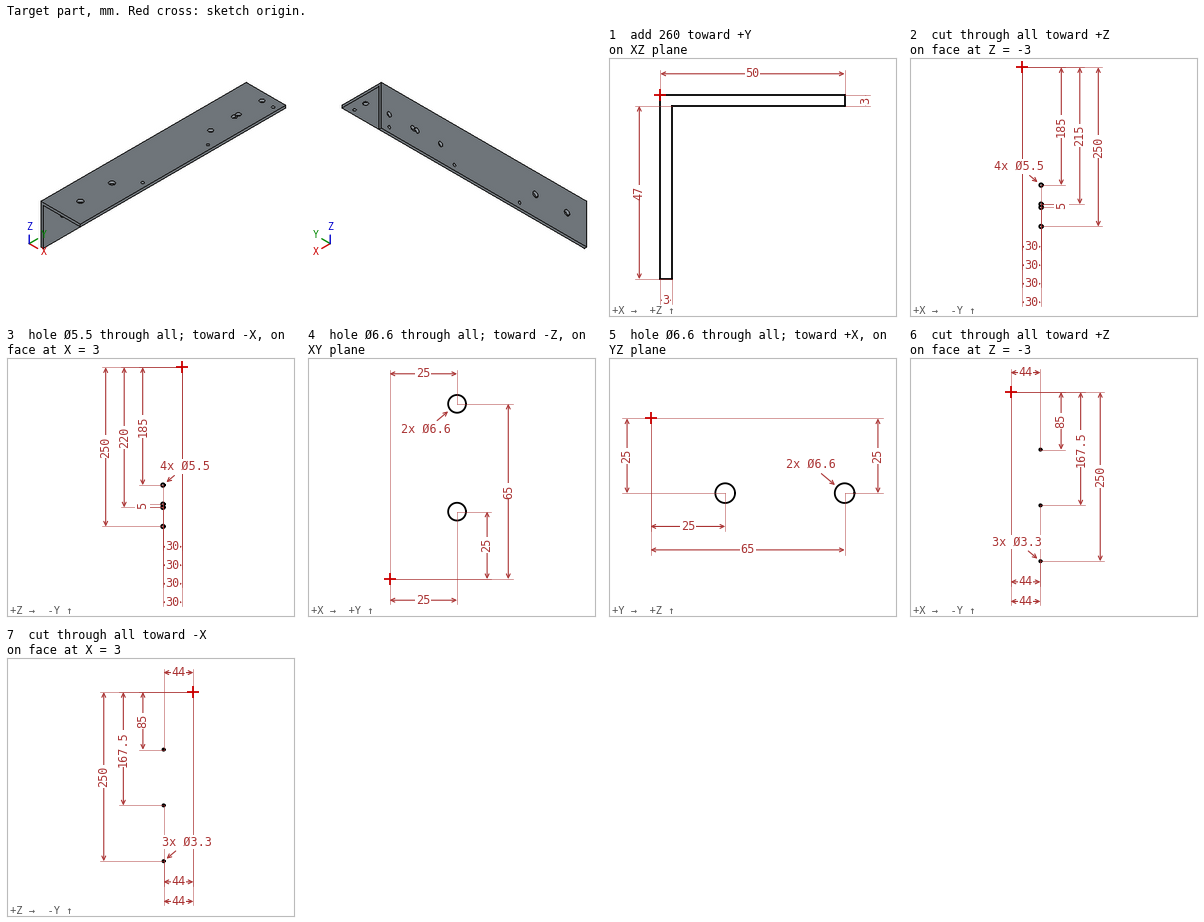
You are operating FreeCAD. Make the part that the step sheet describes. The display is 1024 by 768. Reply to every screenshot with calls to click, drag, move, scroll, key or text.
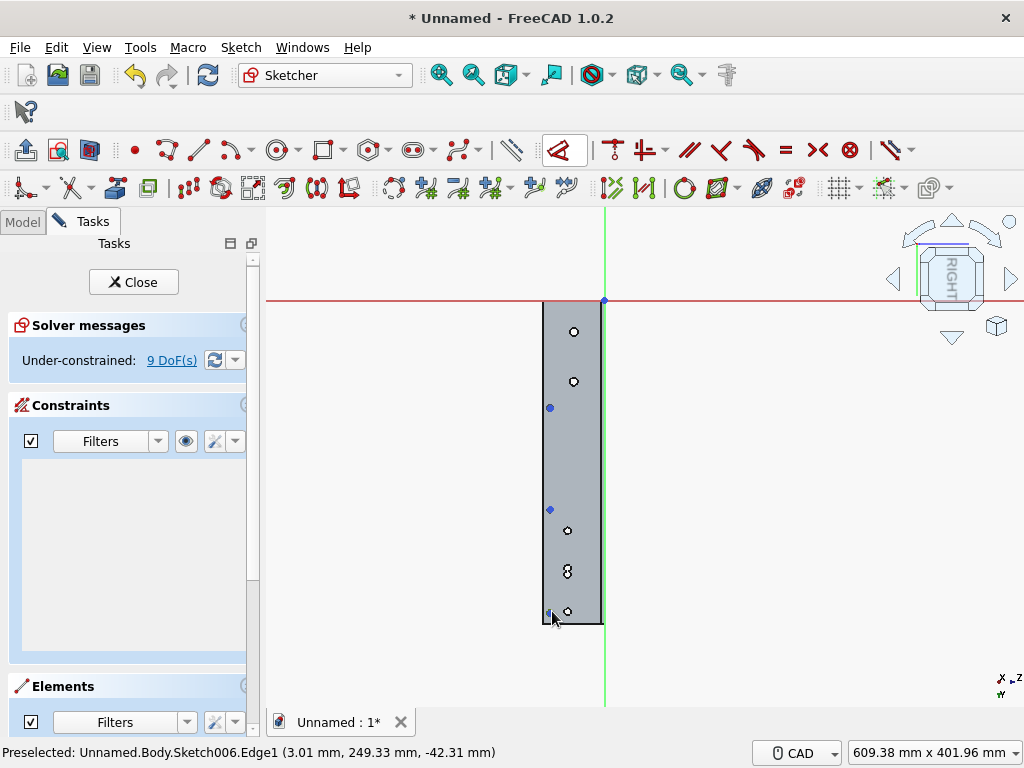
scroll(552, 508, up, 8)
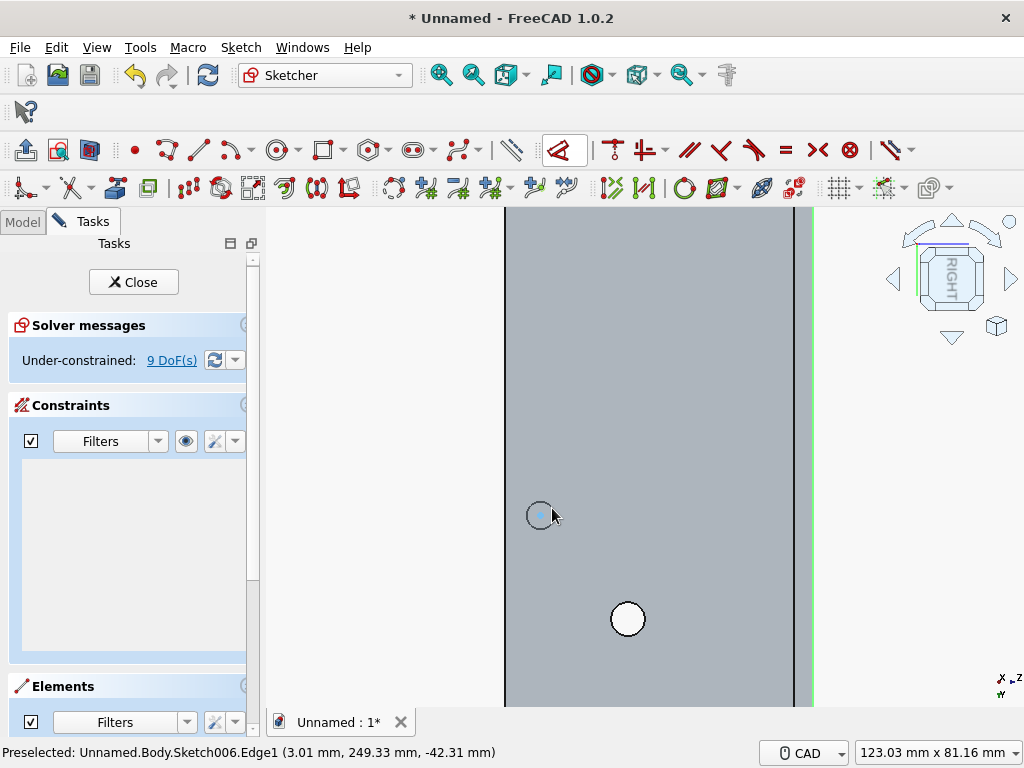
click(550, 506)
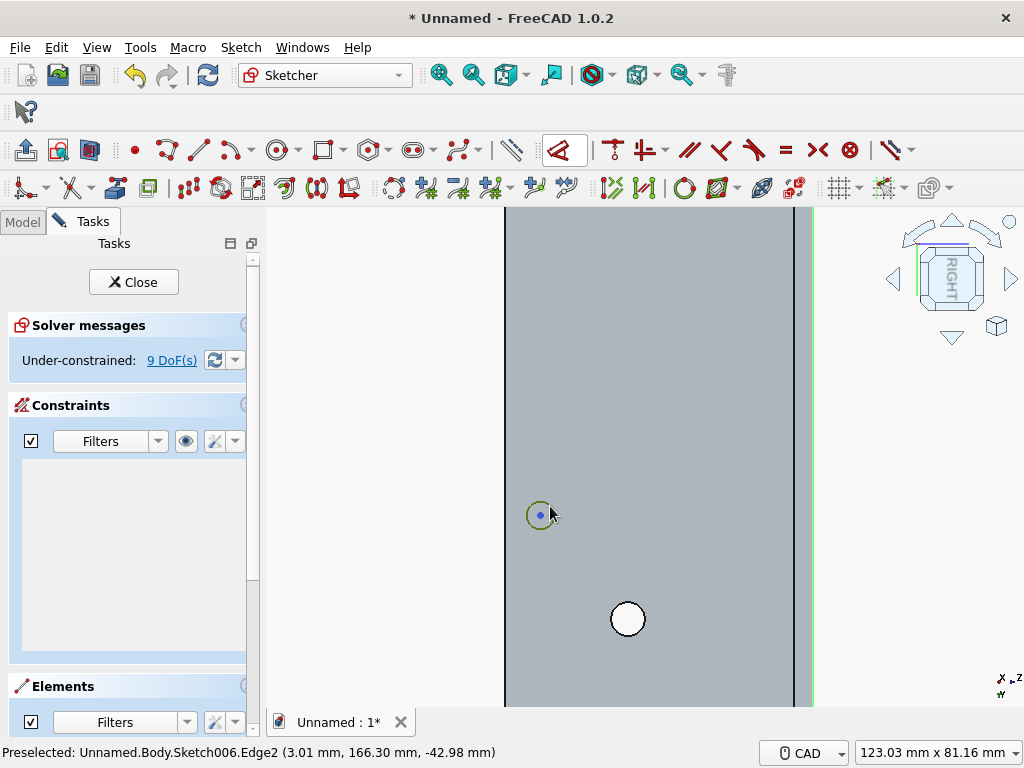
scroll(552, 508, down, 8)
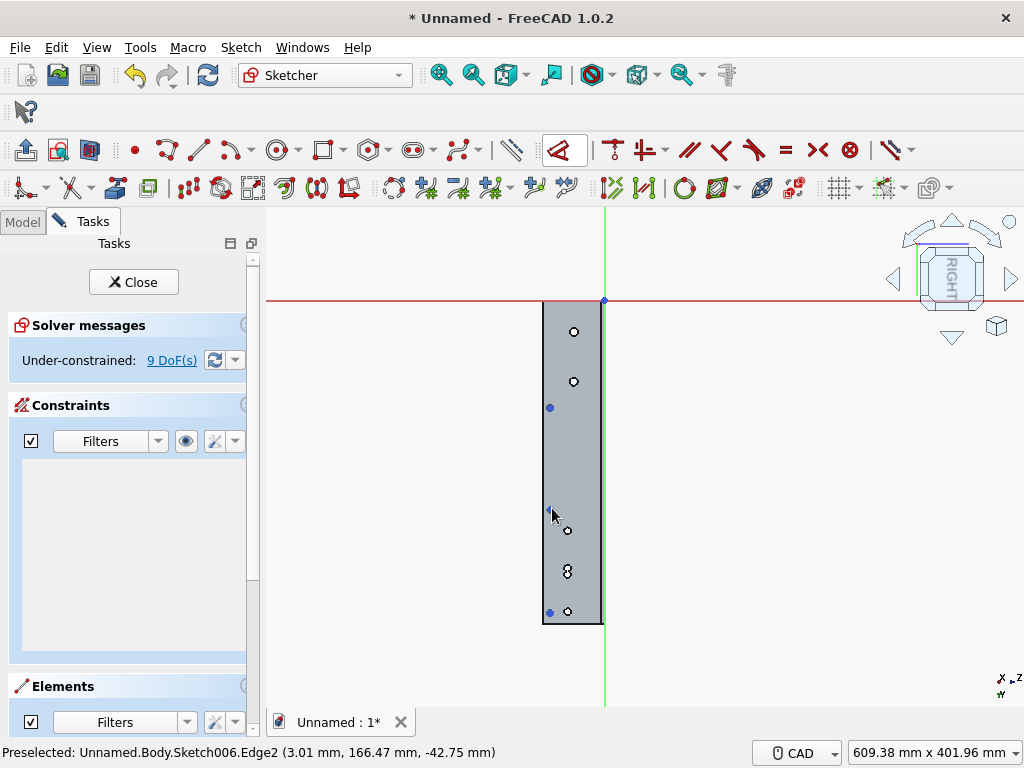
scroll(552, 406, up, 8)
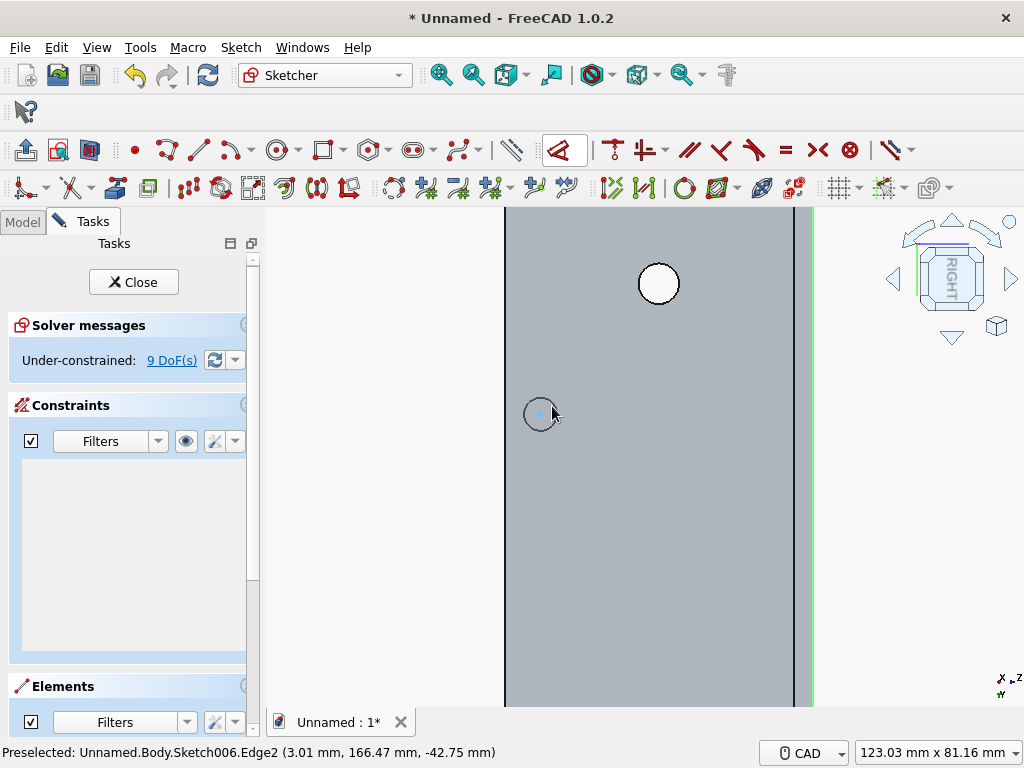
click(552, 403)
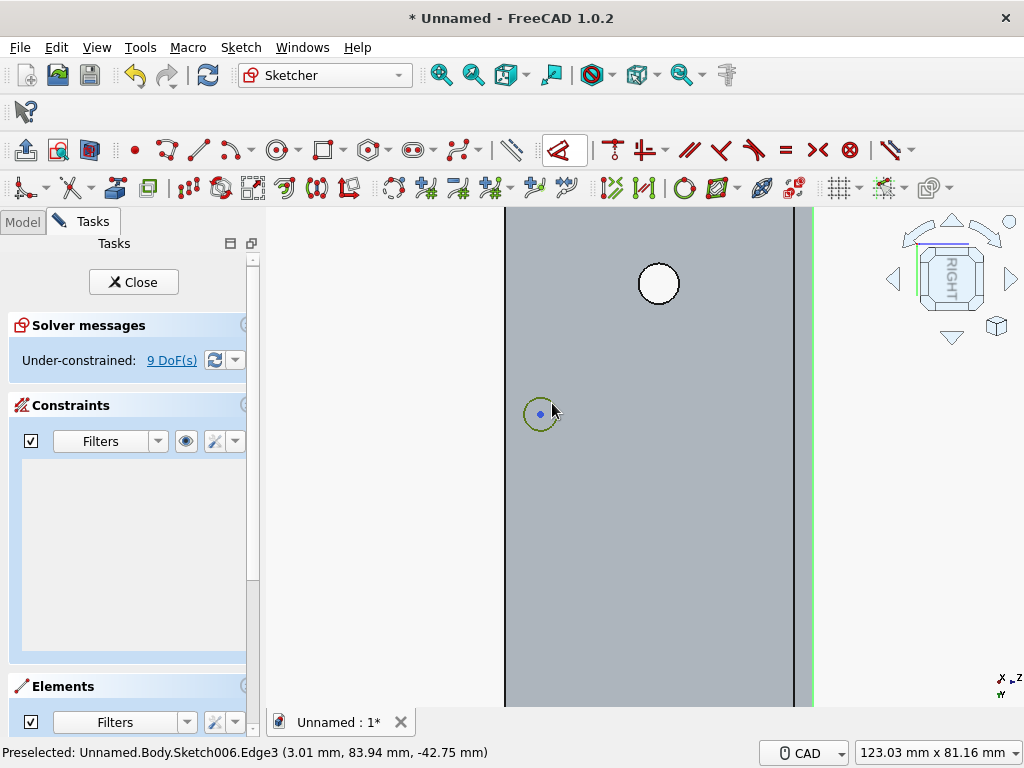
click(786, 150)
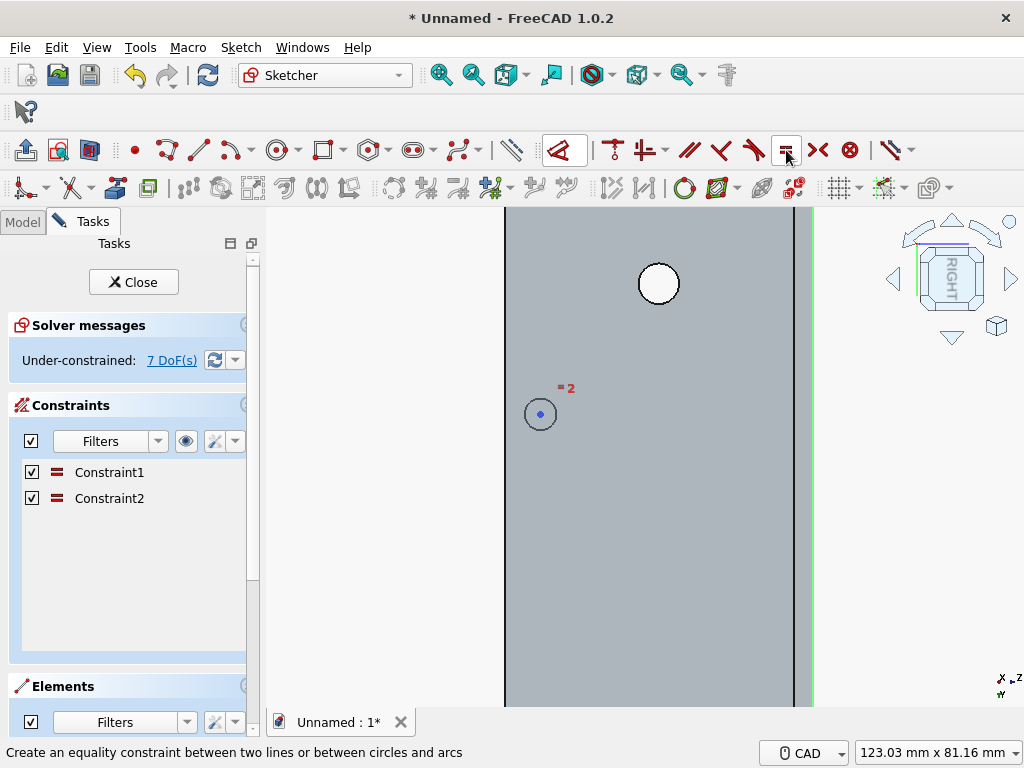
scroll(552, 406, down, 8)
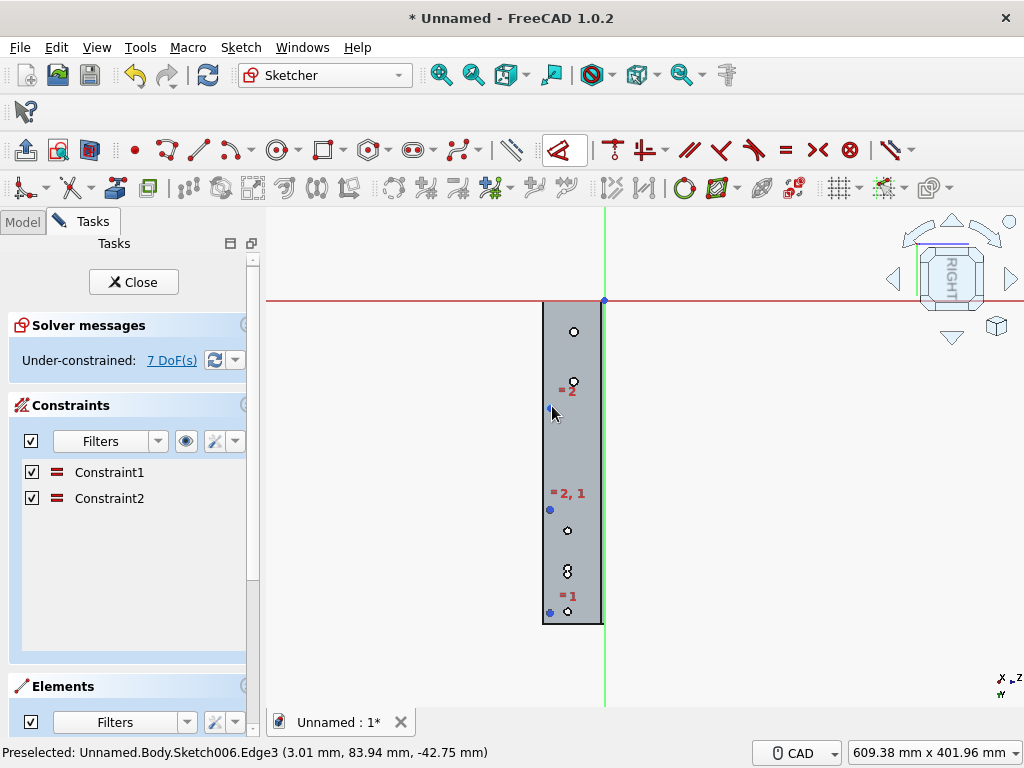
scroll(552, 611, up, 12)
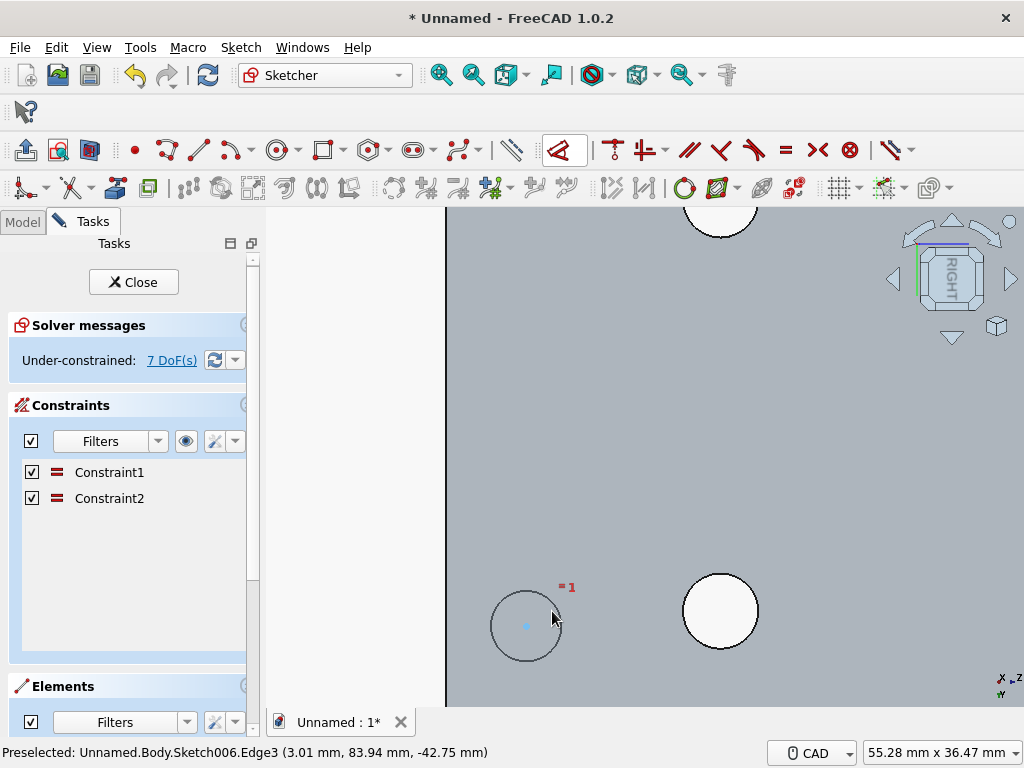
click(551, 601)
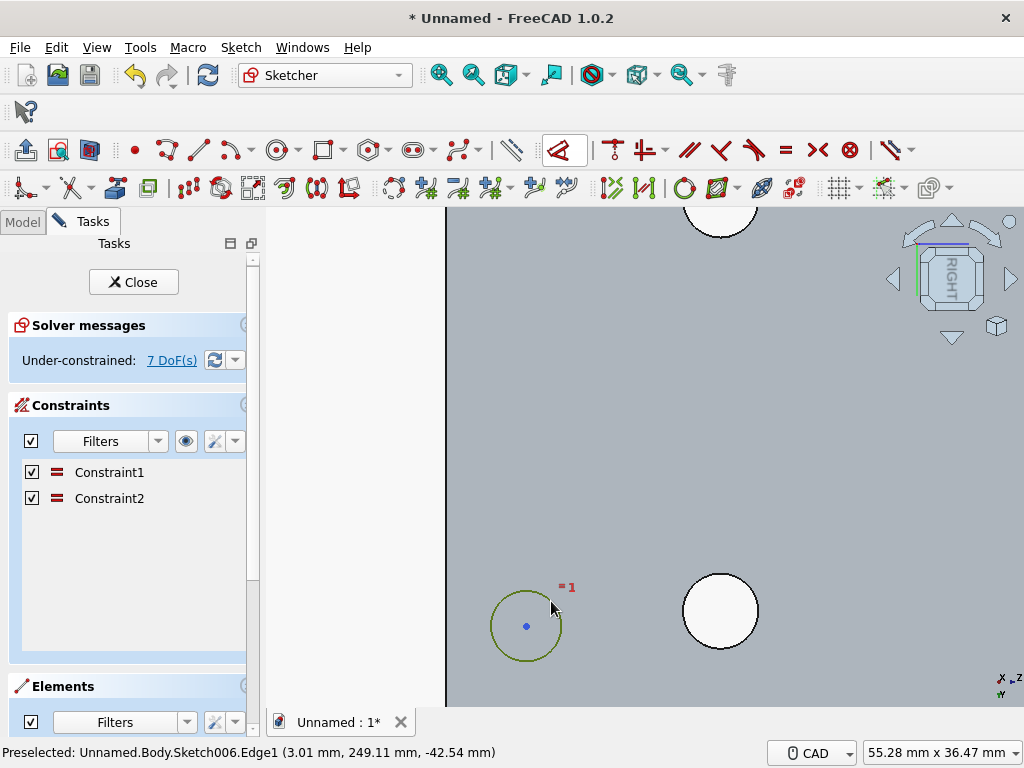
click(582, 150)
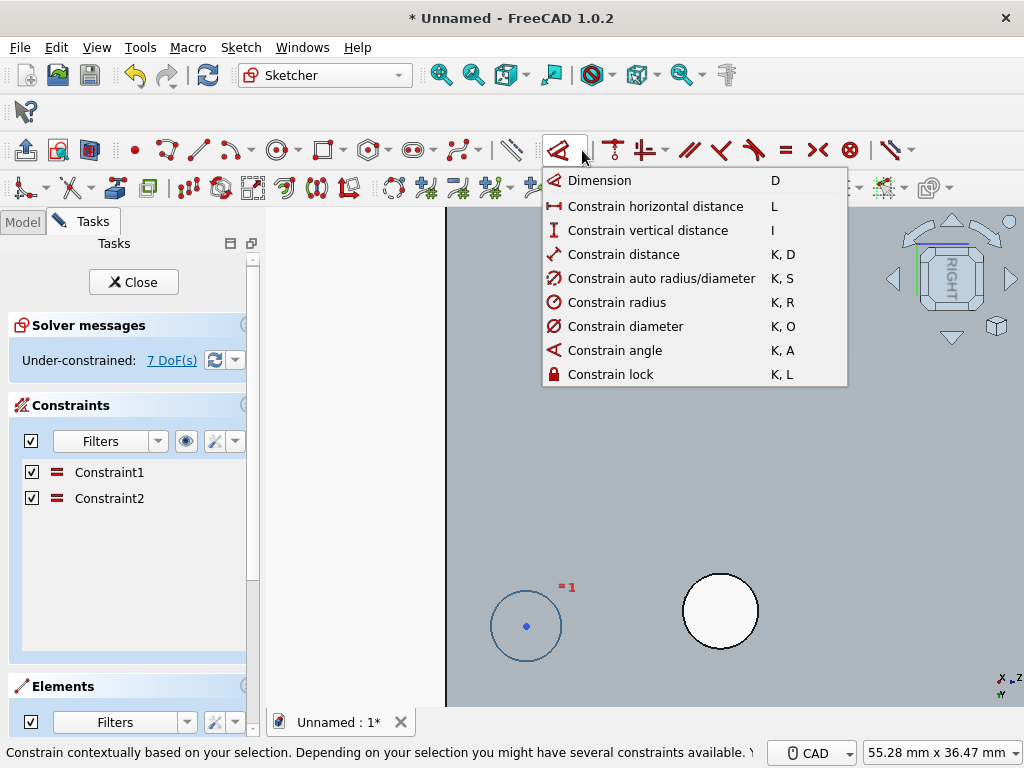
click(695, 326)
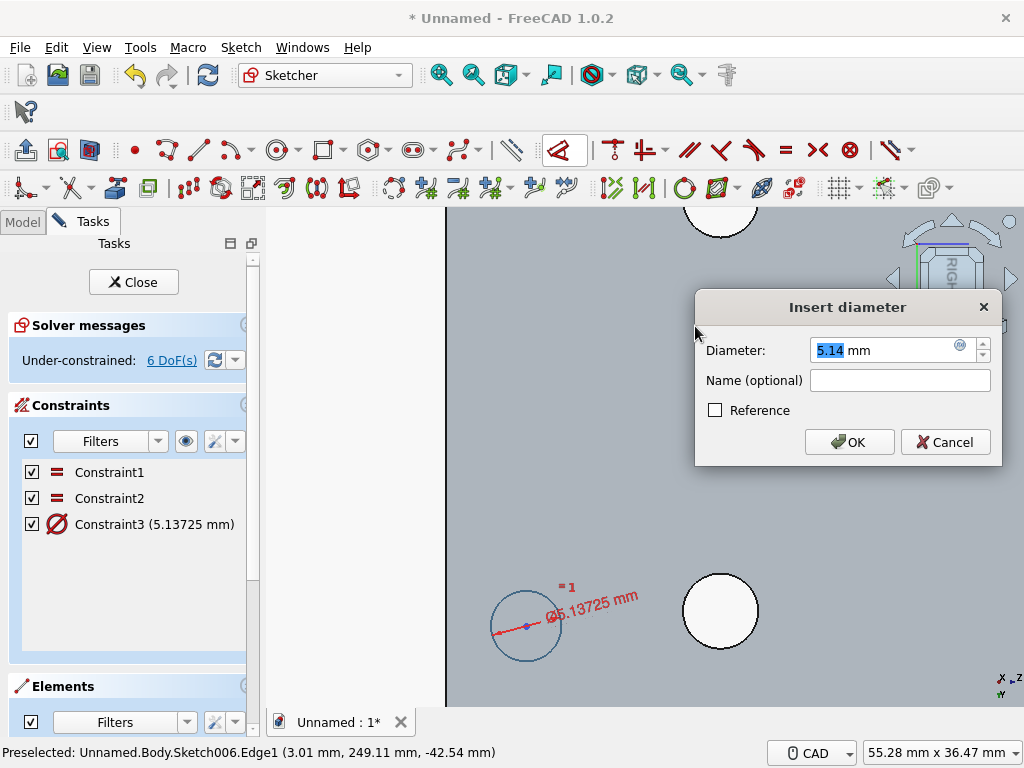
text(3.3)
key(Return)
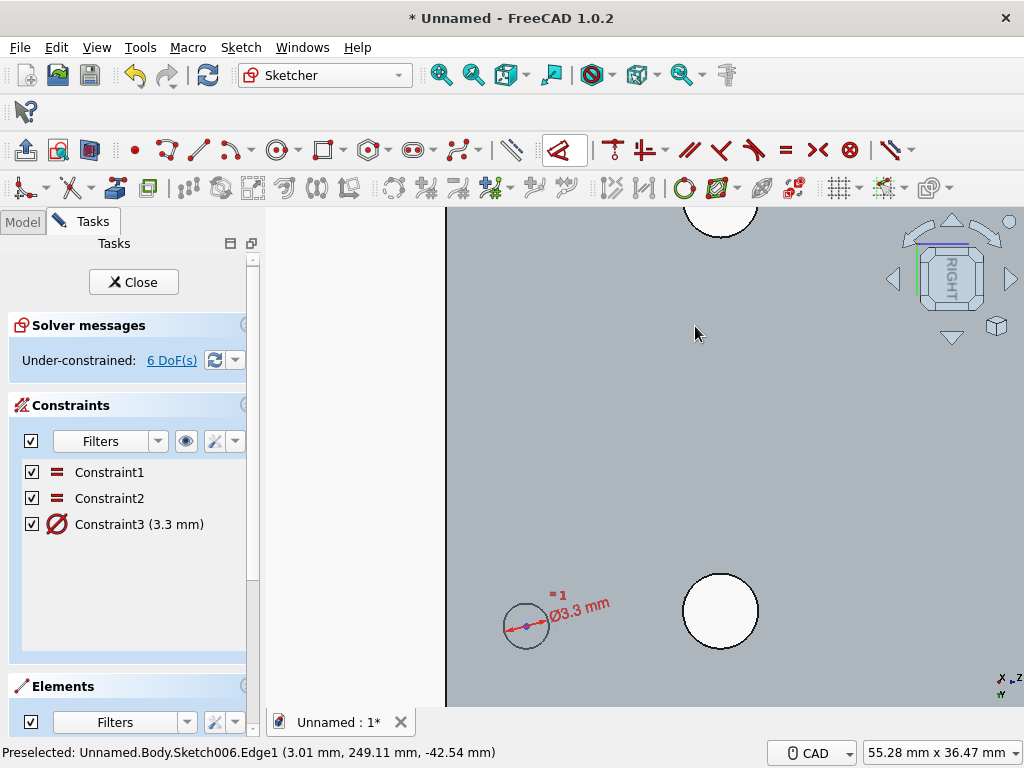
scroll(552, 611, down, 12)